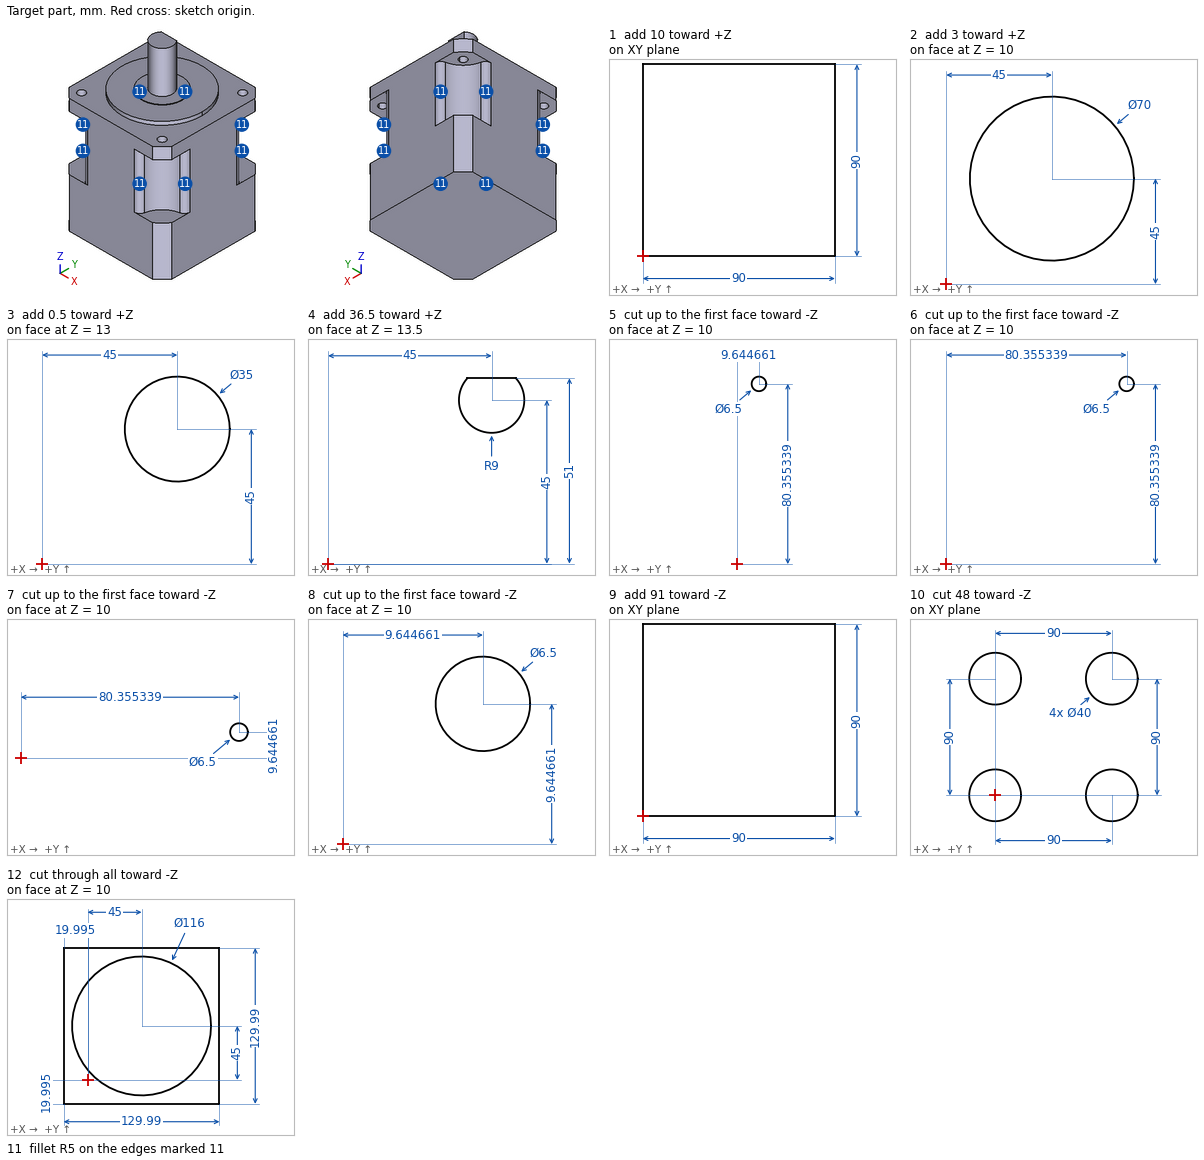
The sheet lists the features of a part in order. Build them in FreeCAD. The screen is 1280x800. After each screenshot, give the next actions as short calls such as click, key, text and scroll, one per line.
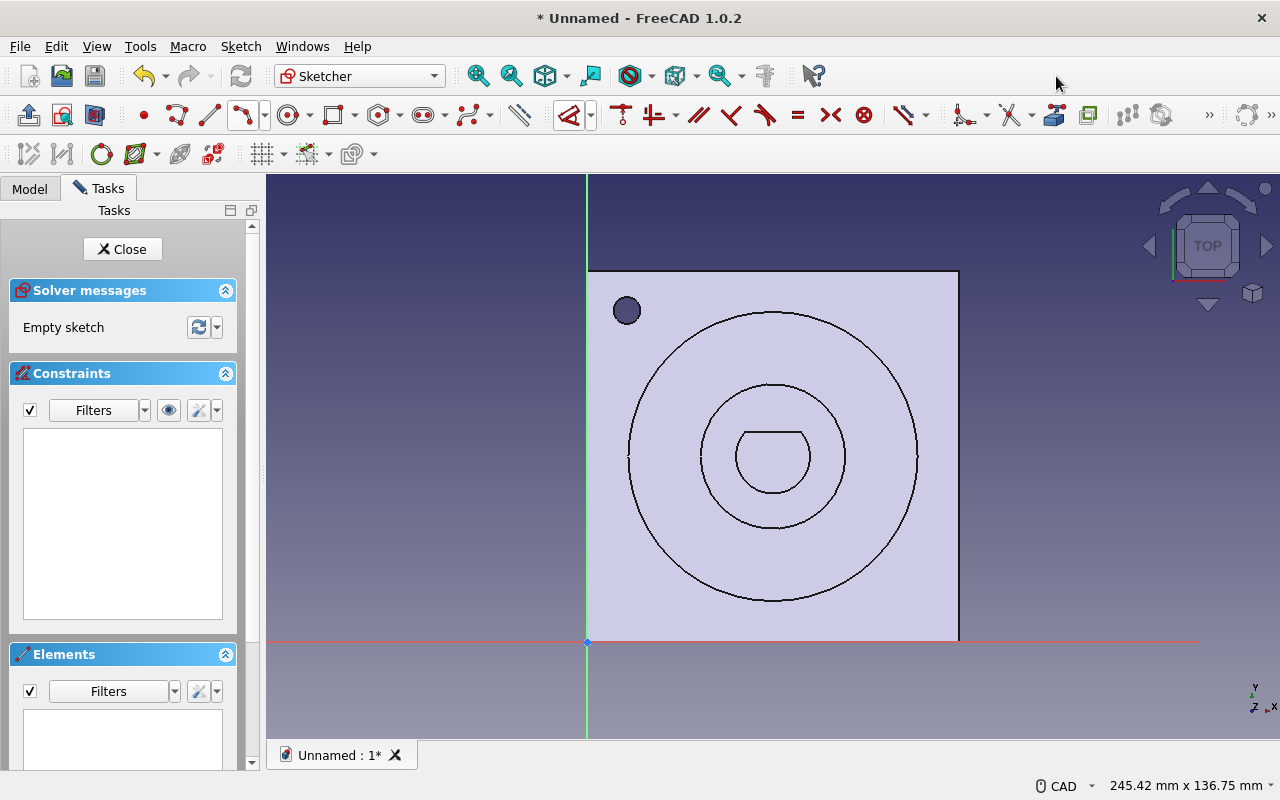
scroll(936, 299, up, 13)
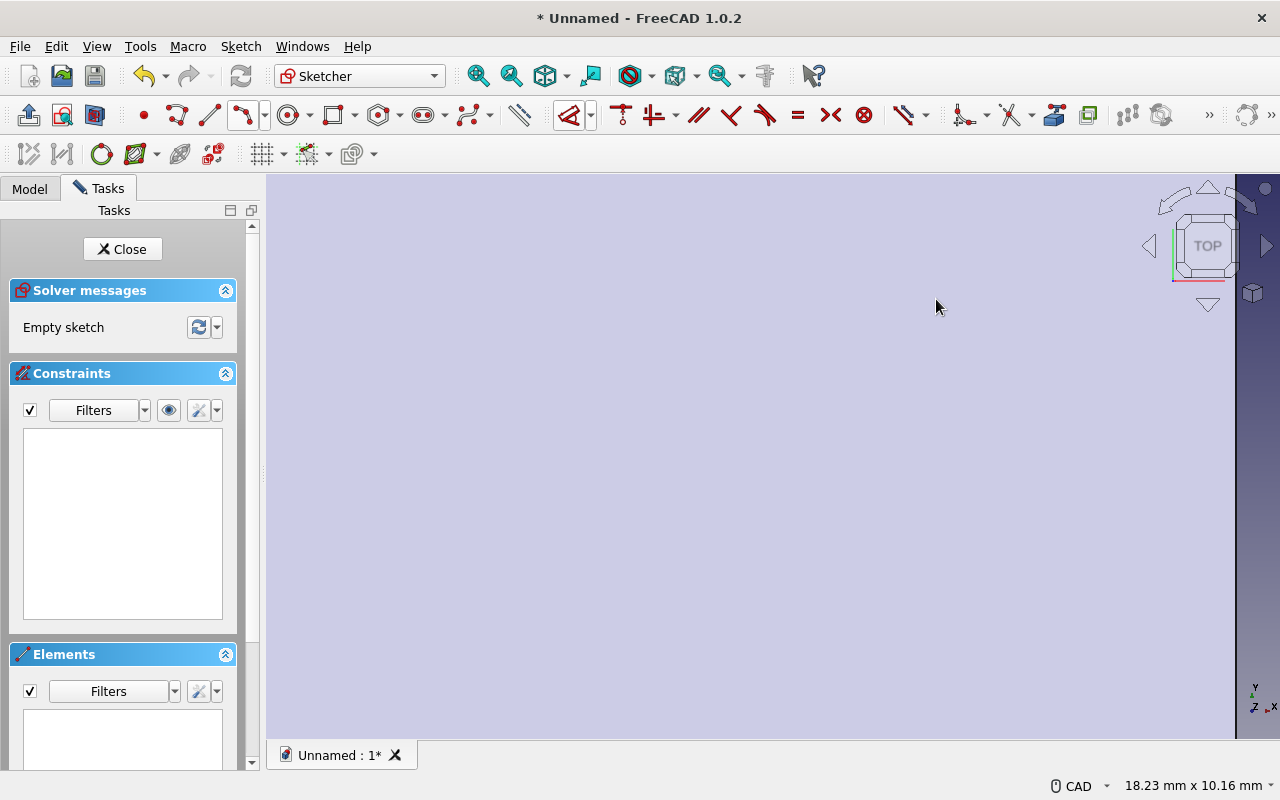
key(g)
key(c)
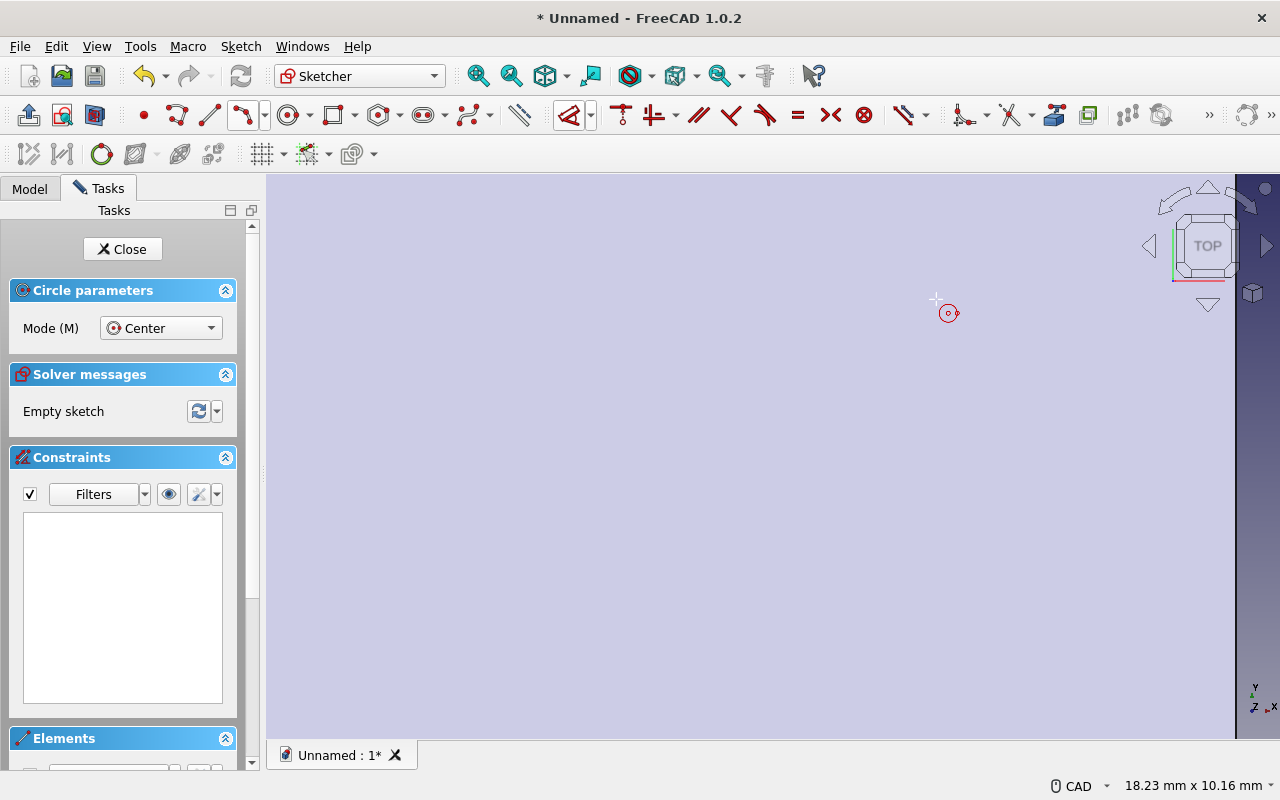
click(700, 450)
move(828, 322)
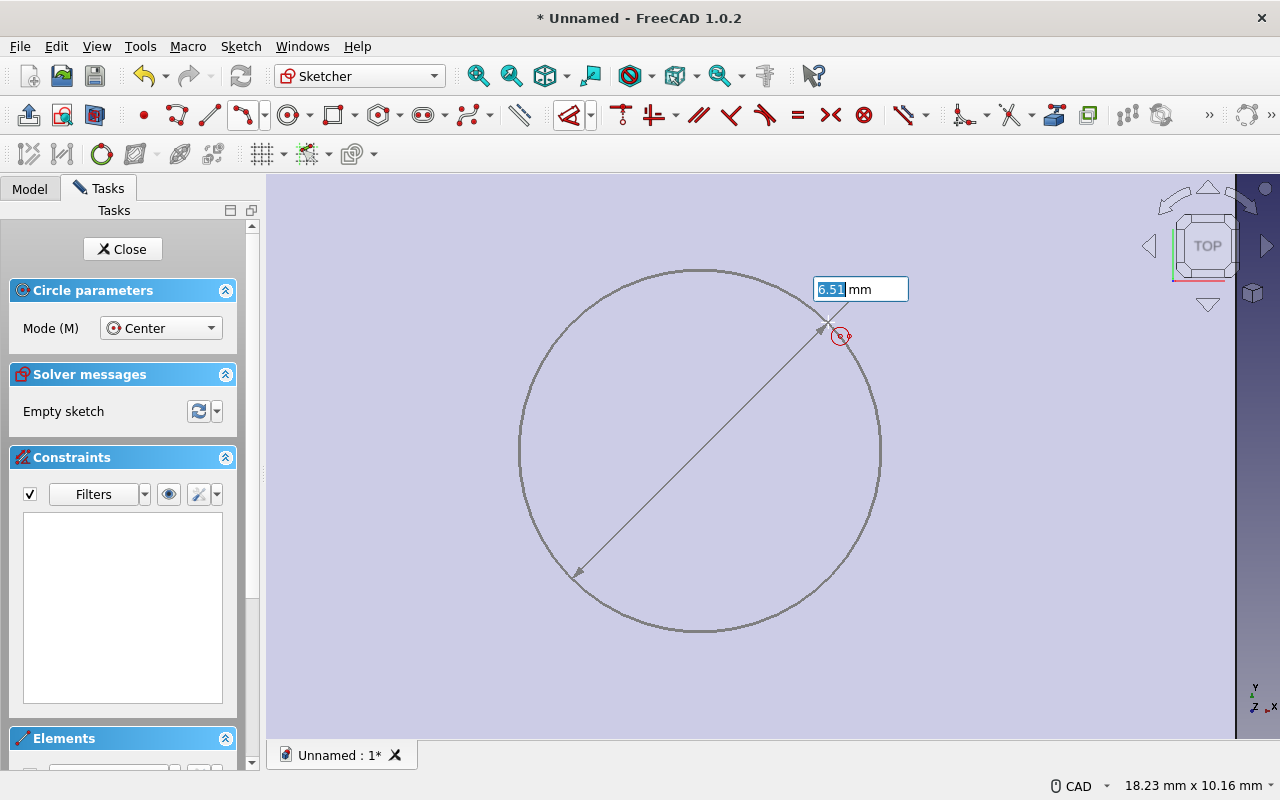
text(6.5)
key(Return)
key(Escape)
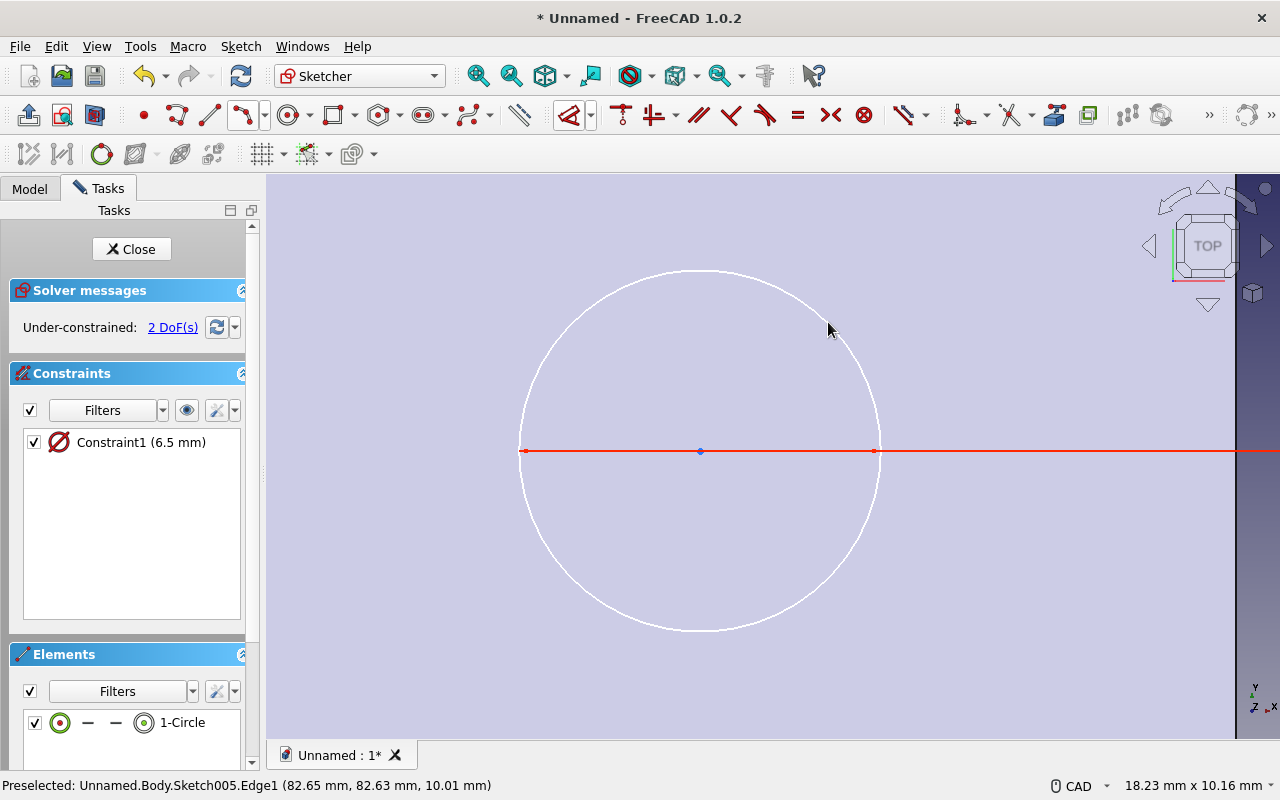
click(700, 451)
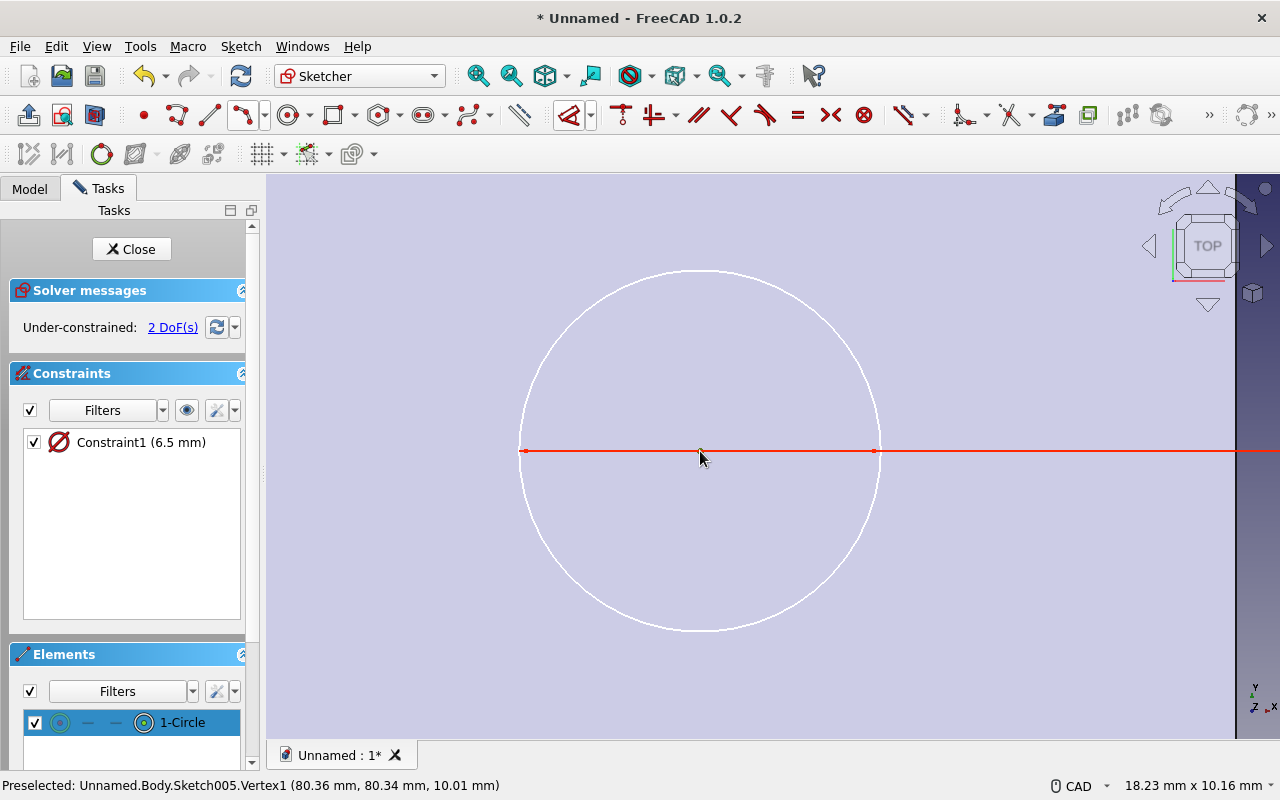
click(590, 116)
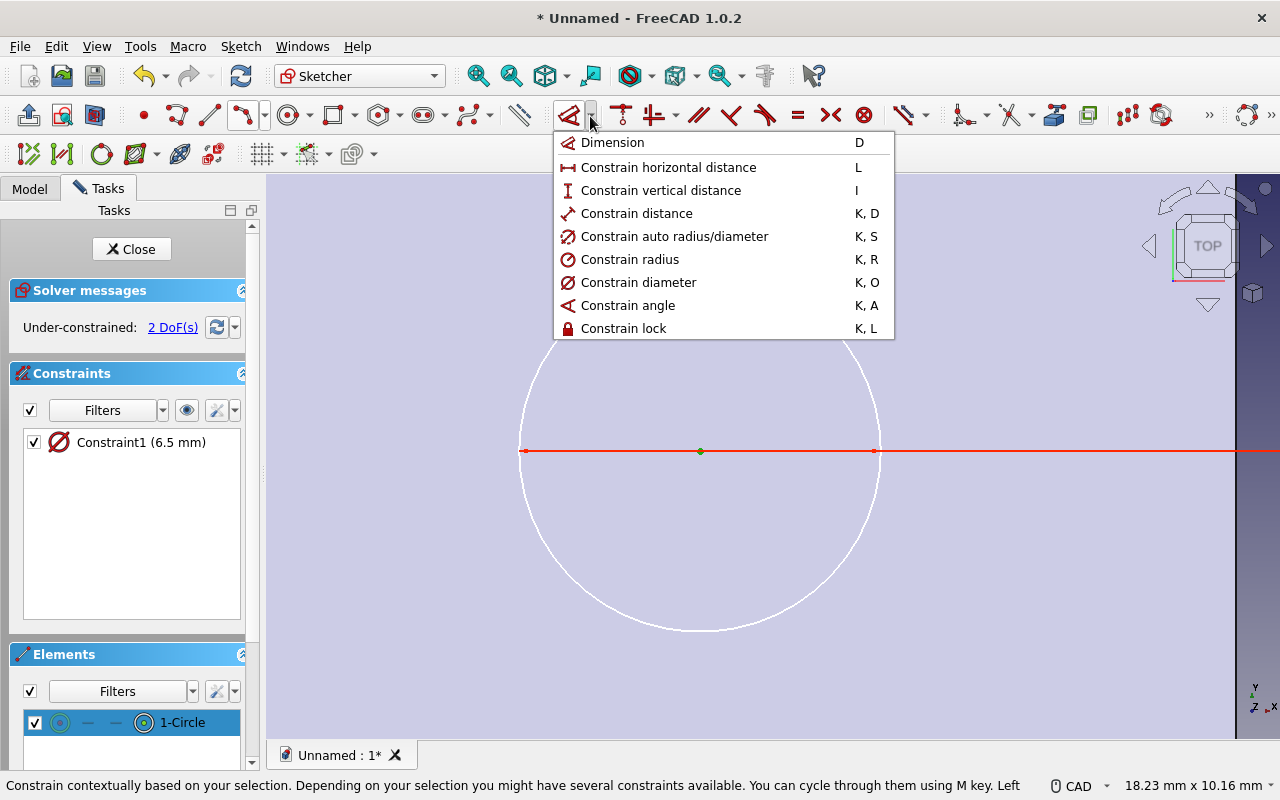
click(724, 168)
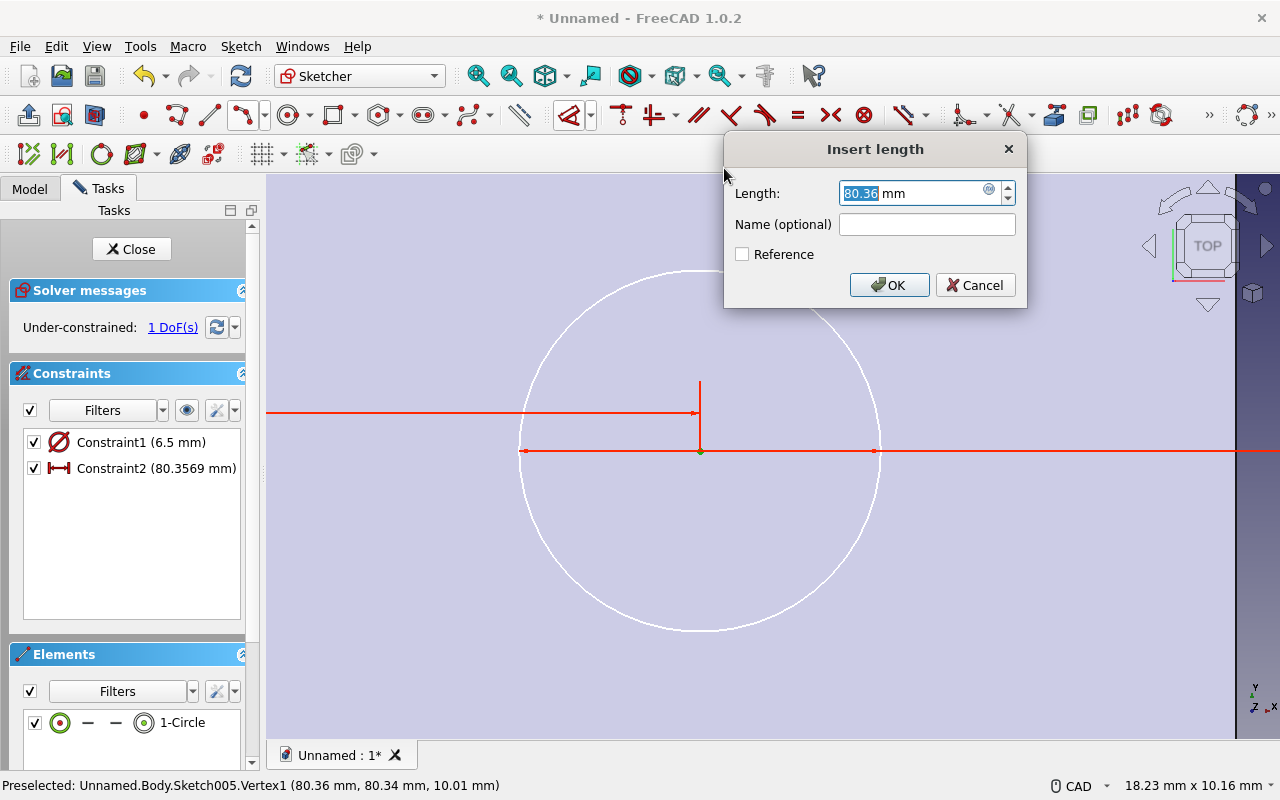
text(80.355339)
key(Return)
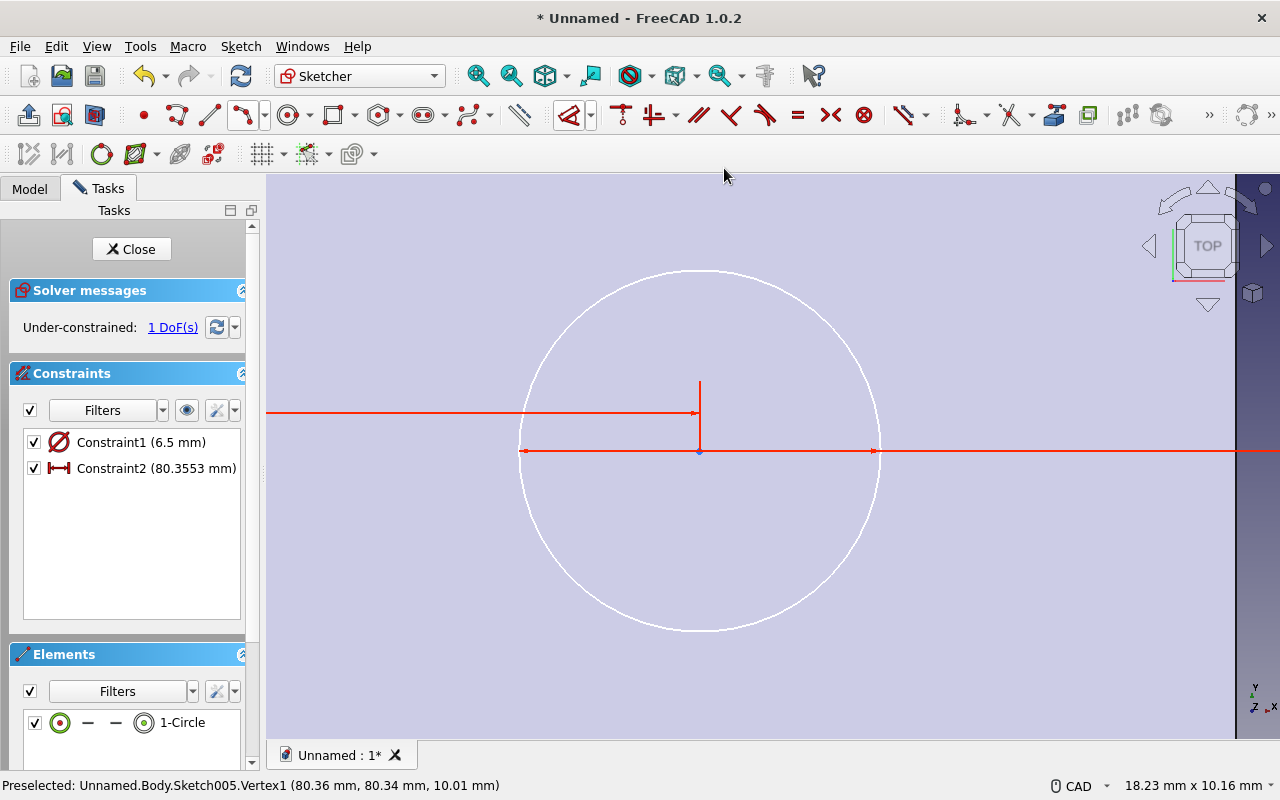
click(700, 451)